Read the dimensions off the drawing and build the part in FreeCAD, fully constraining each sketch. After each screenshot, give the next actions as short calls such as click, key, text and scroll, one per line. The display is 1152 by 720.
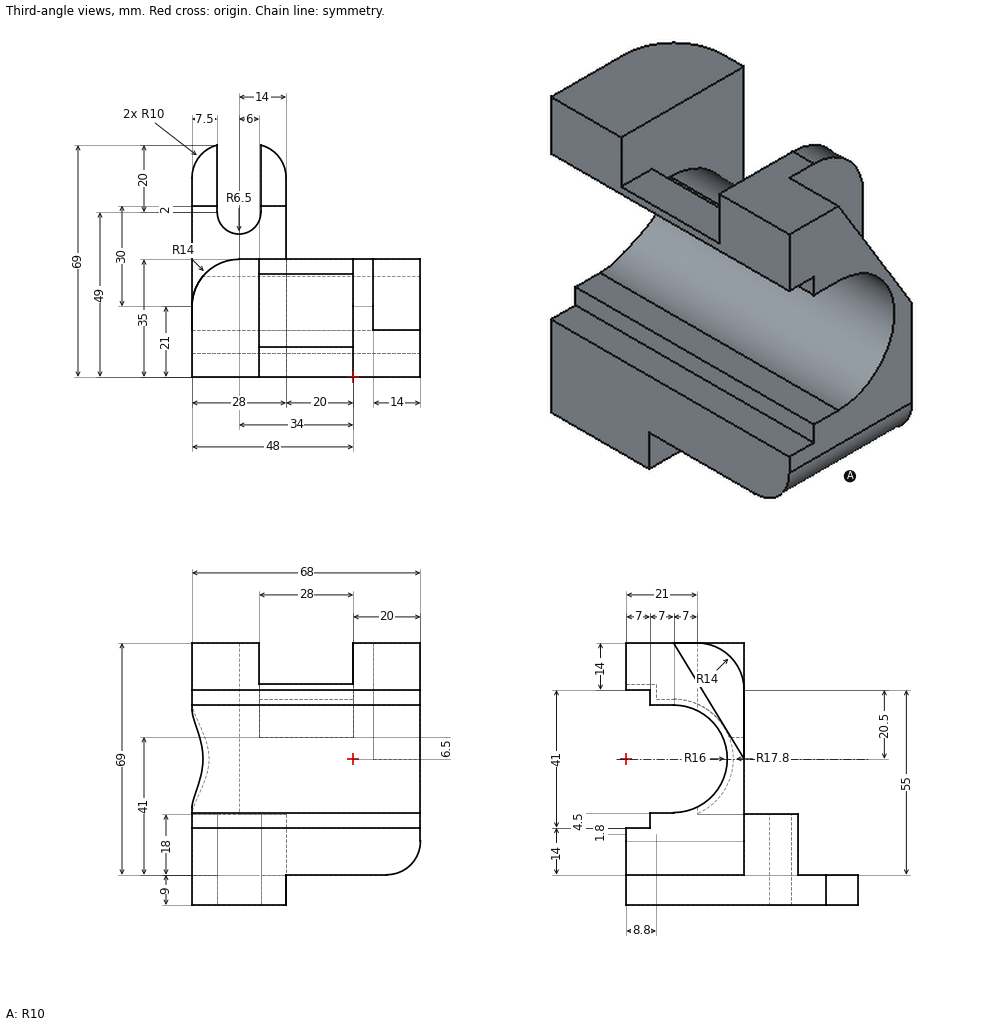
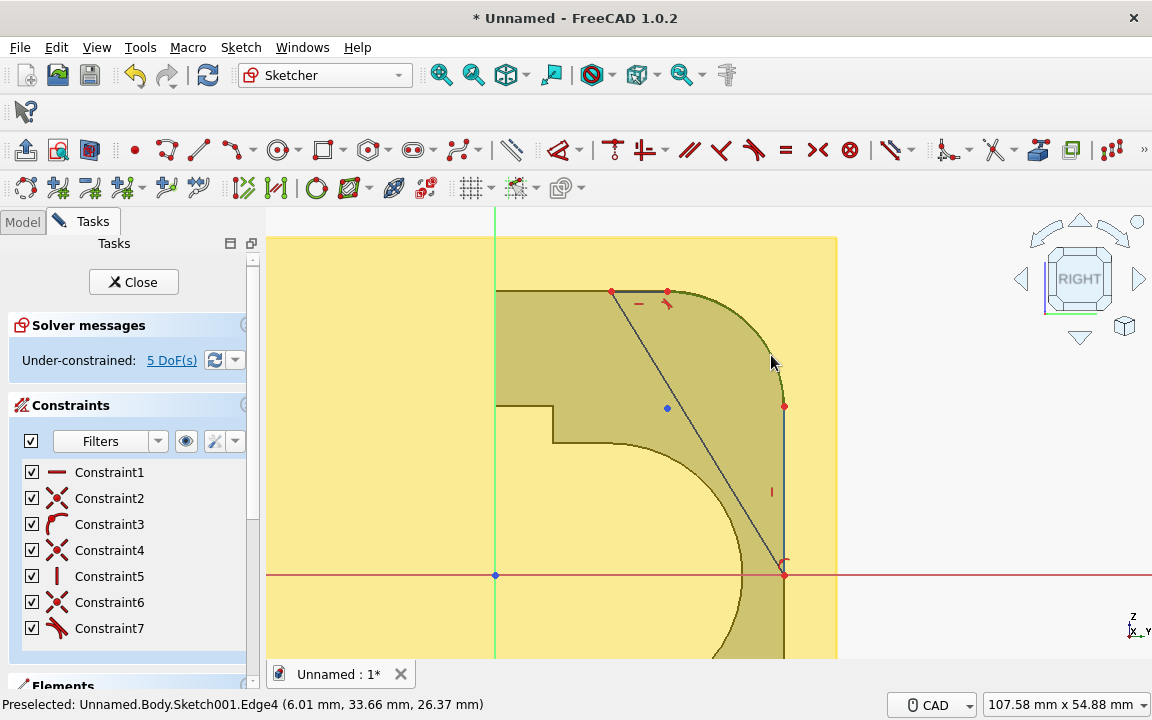
click(754, 150)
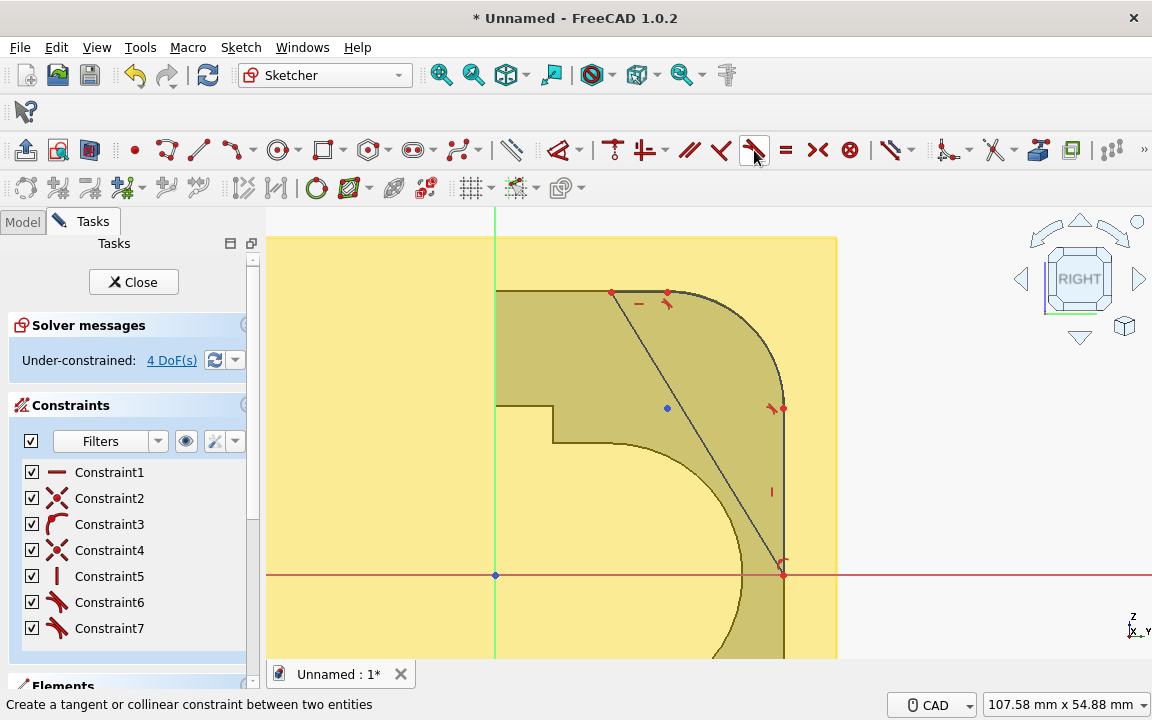
key(d)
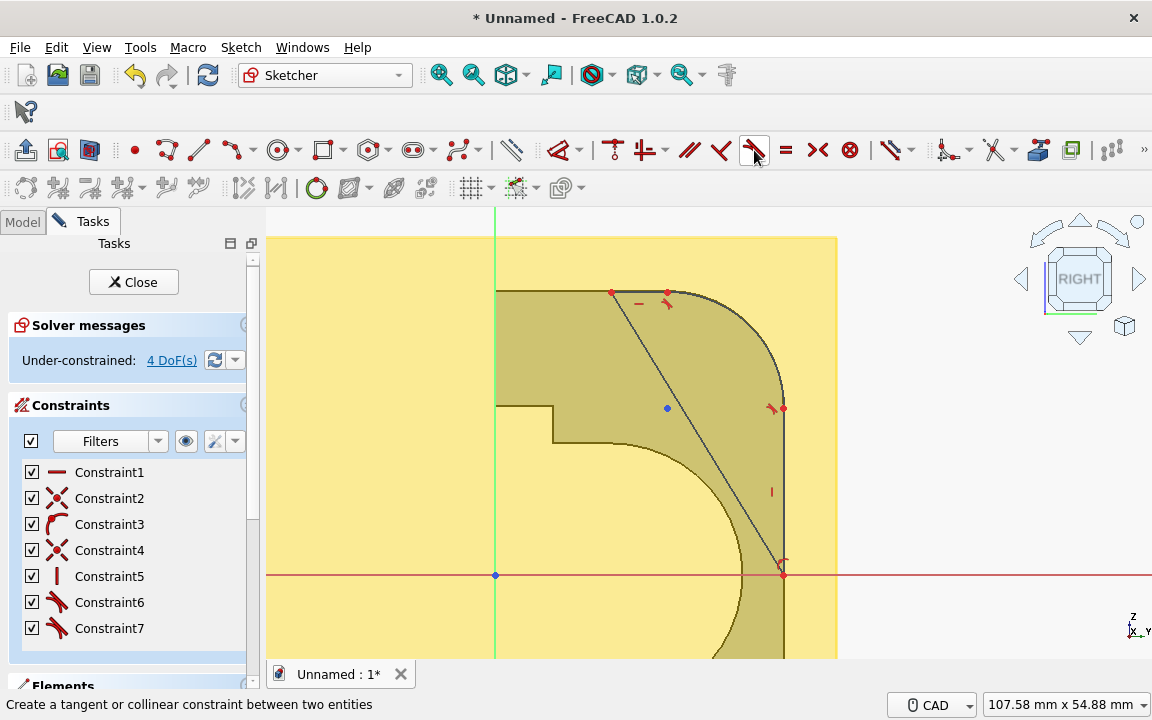
click(771, 355)
click(799, 340)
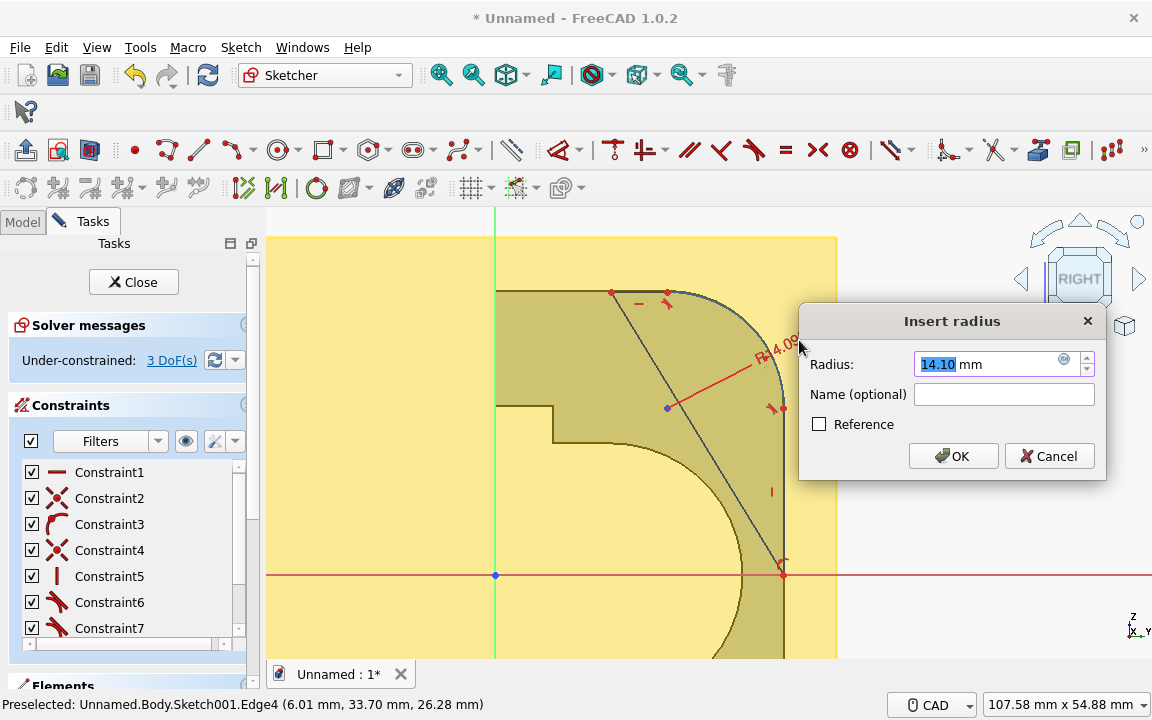
text(14)
key(Return)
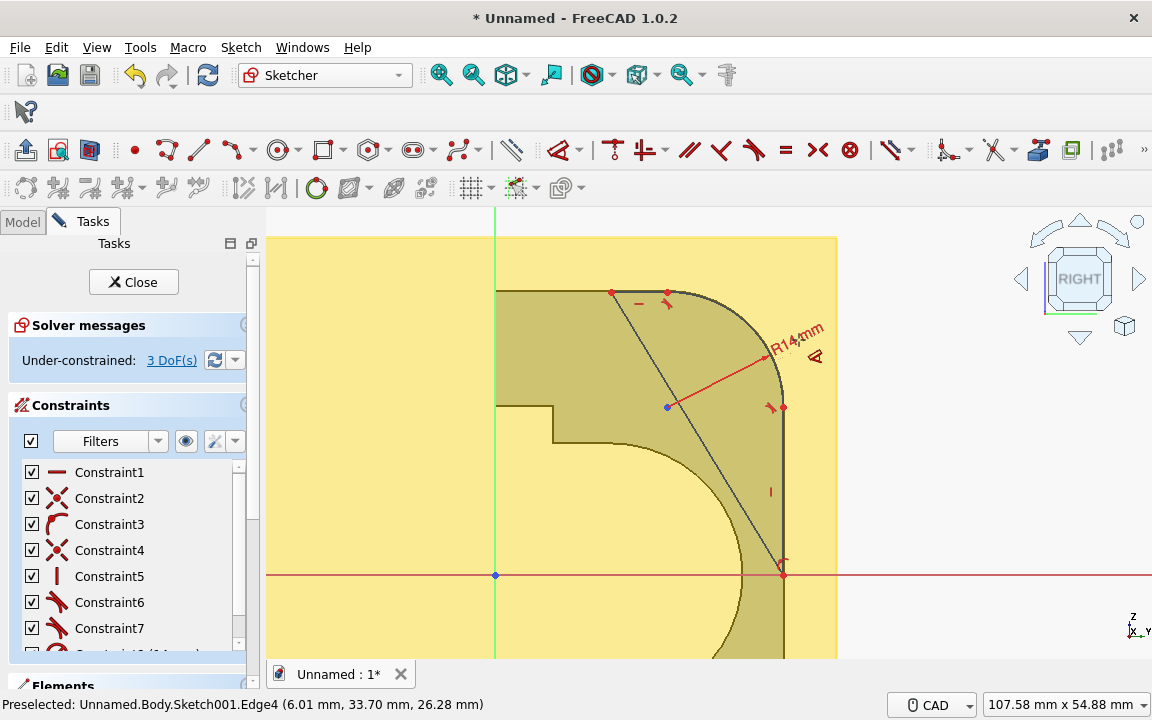
click(651, 292)
click(639, 258)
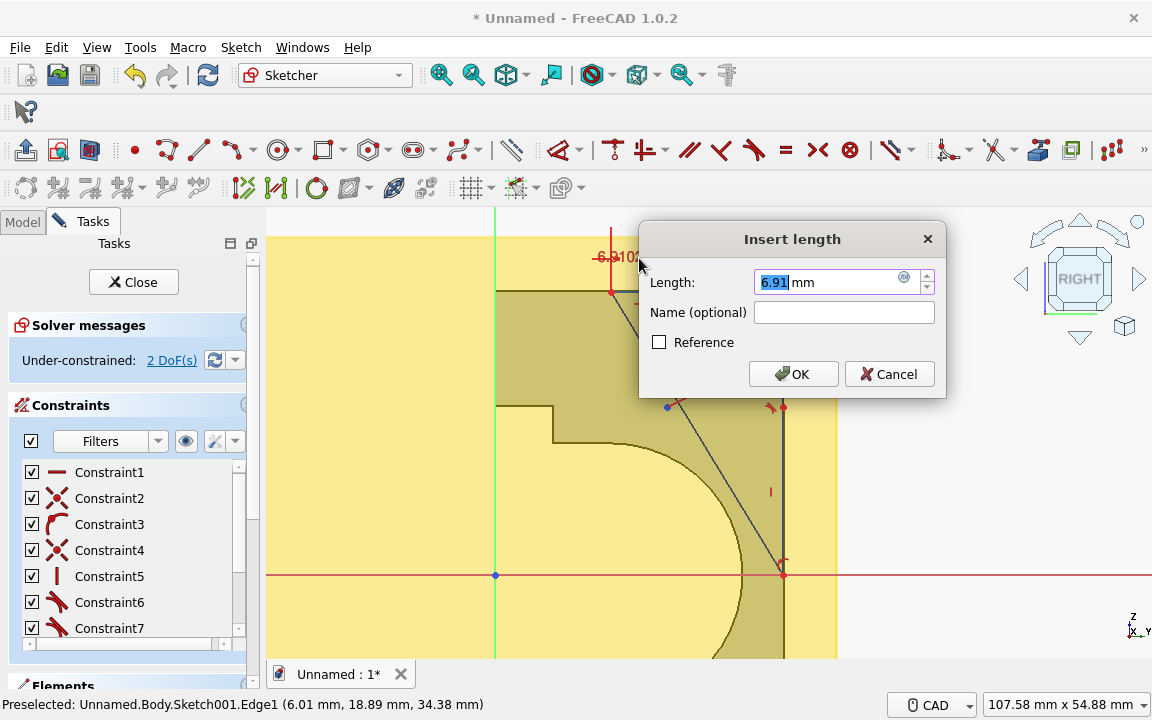
text(7)
key(Return)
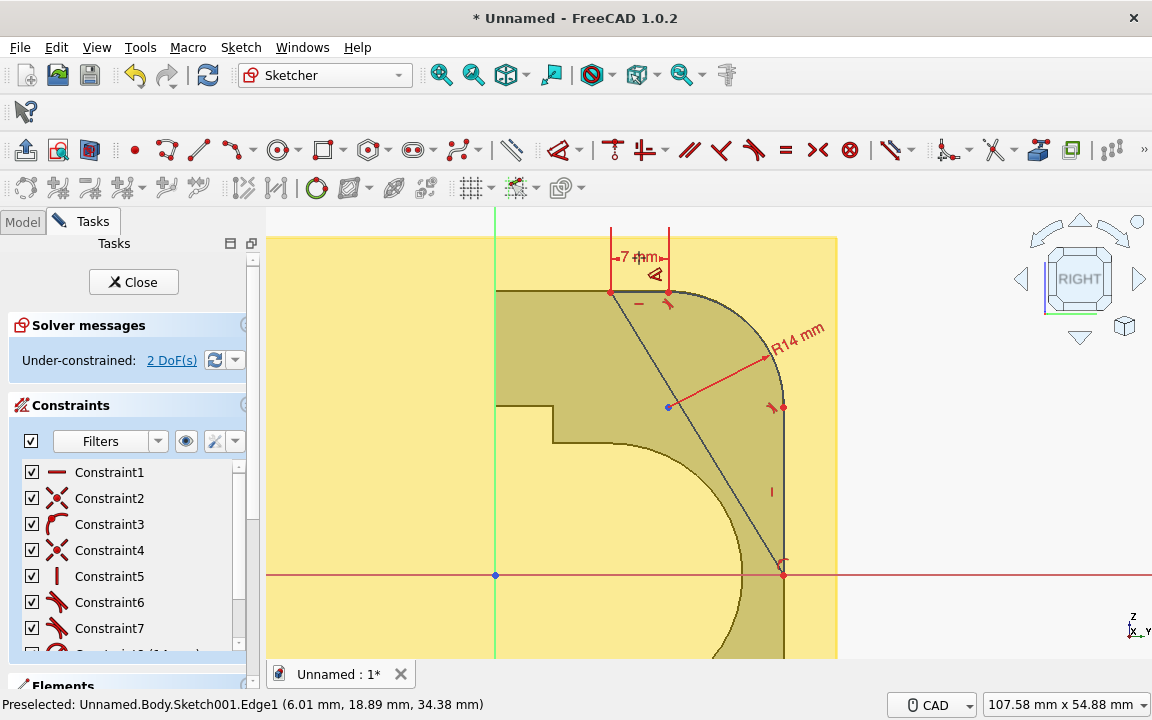
click(669, 292)
click(582, 609)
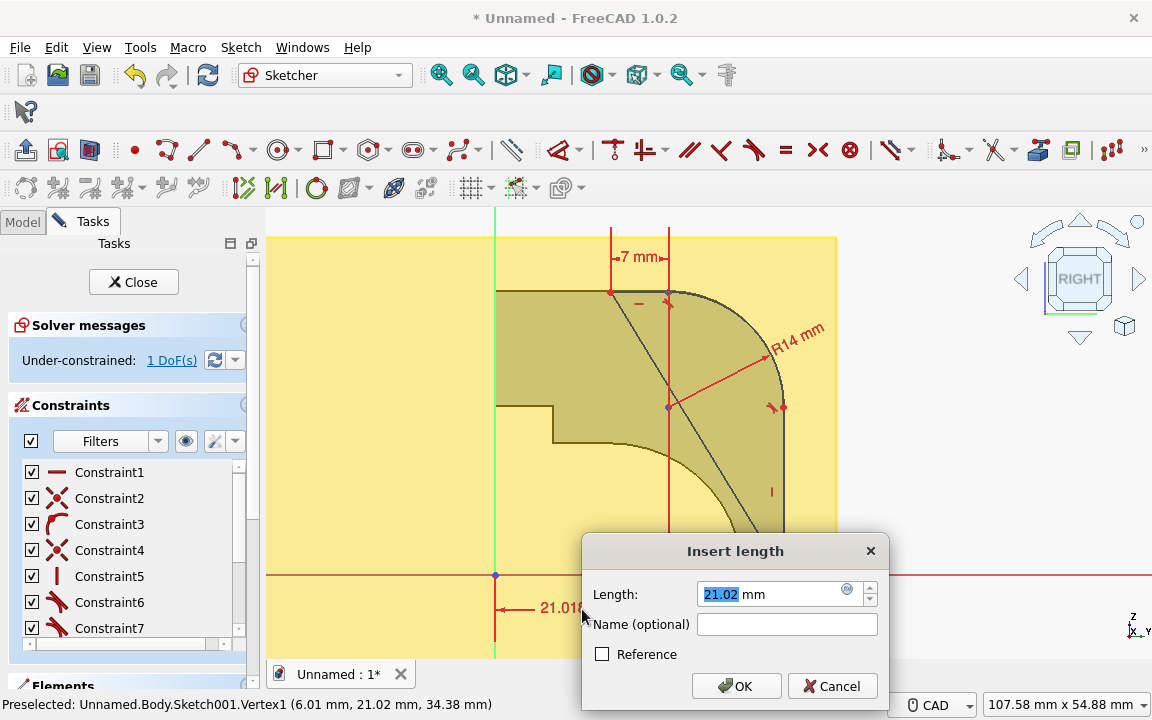
text(21)
key(Return)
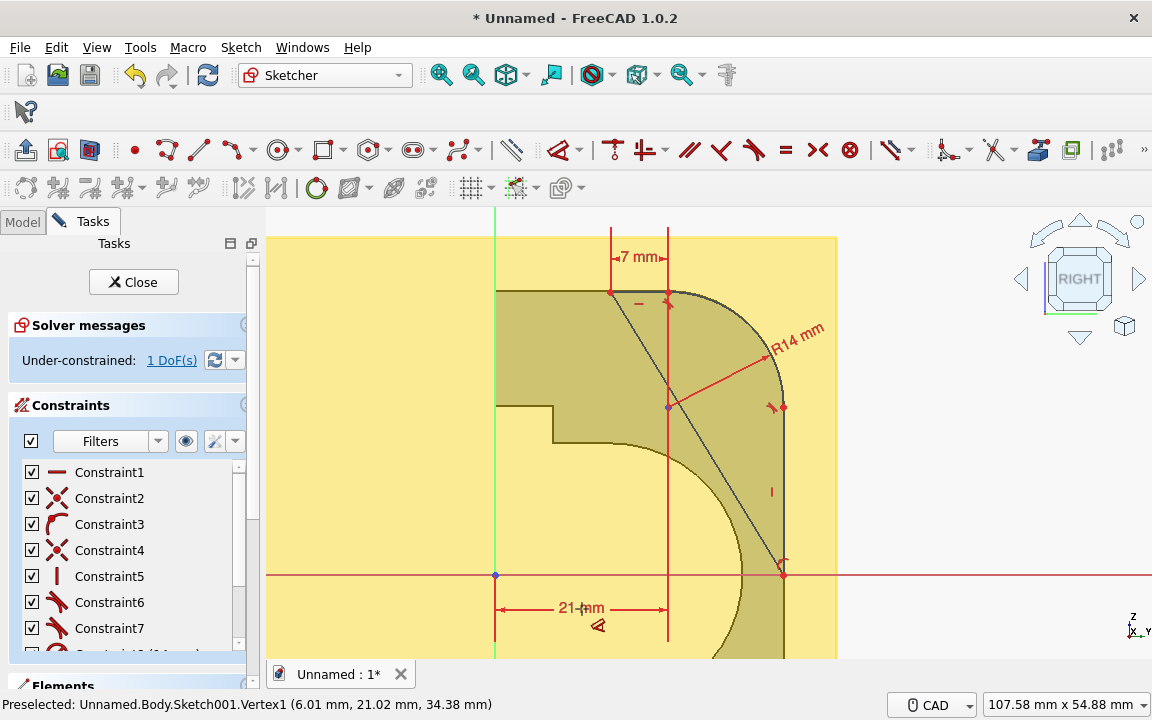
click(784, 525)
click(818, 491)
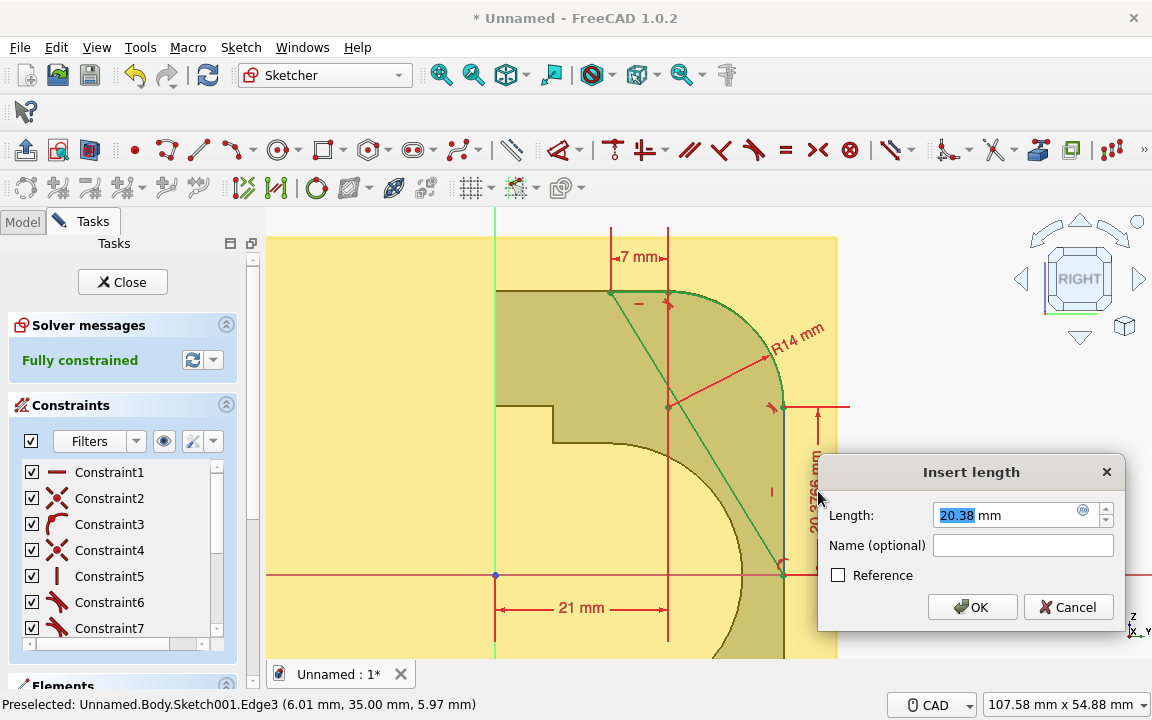
text(20.5)
key(Return)
key(Escape)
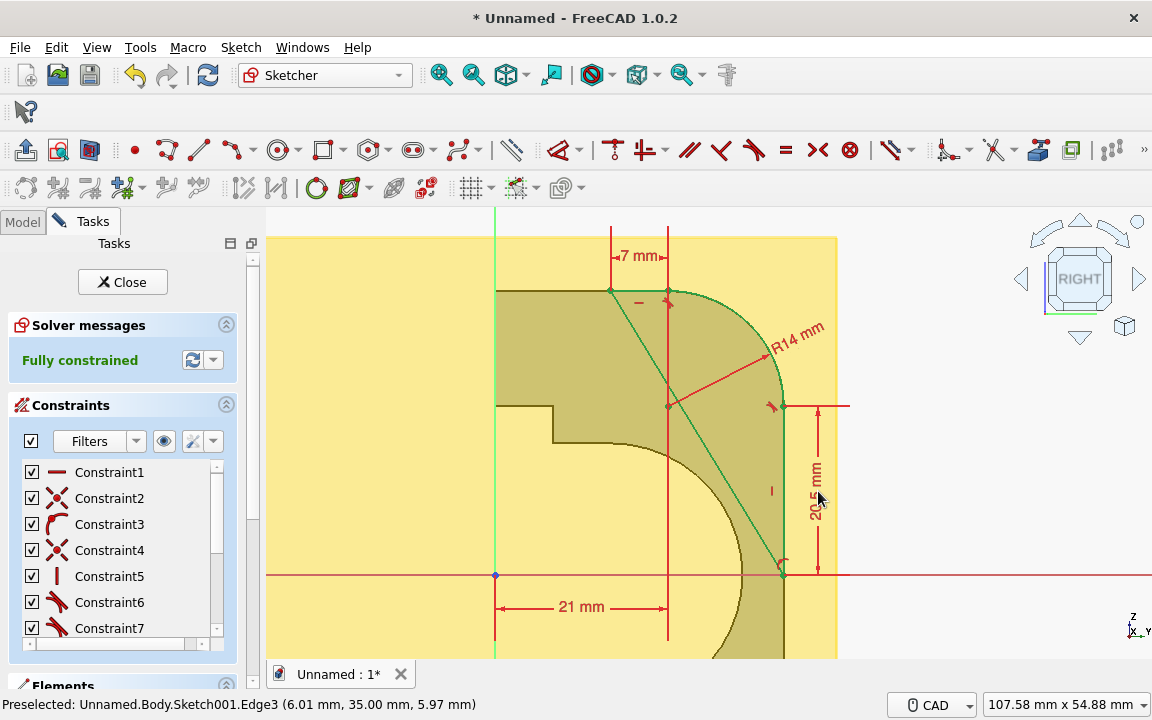
click(123, 282)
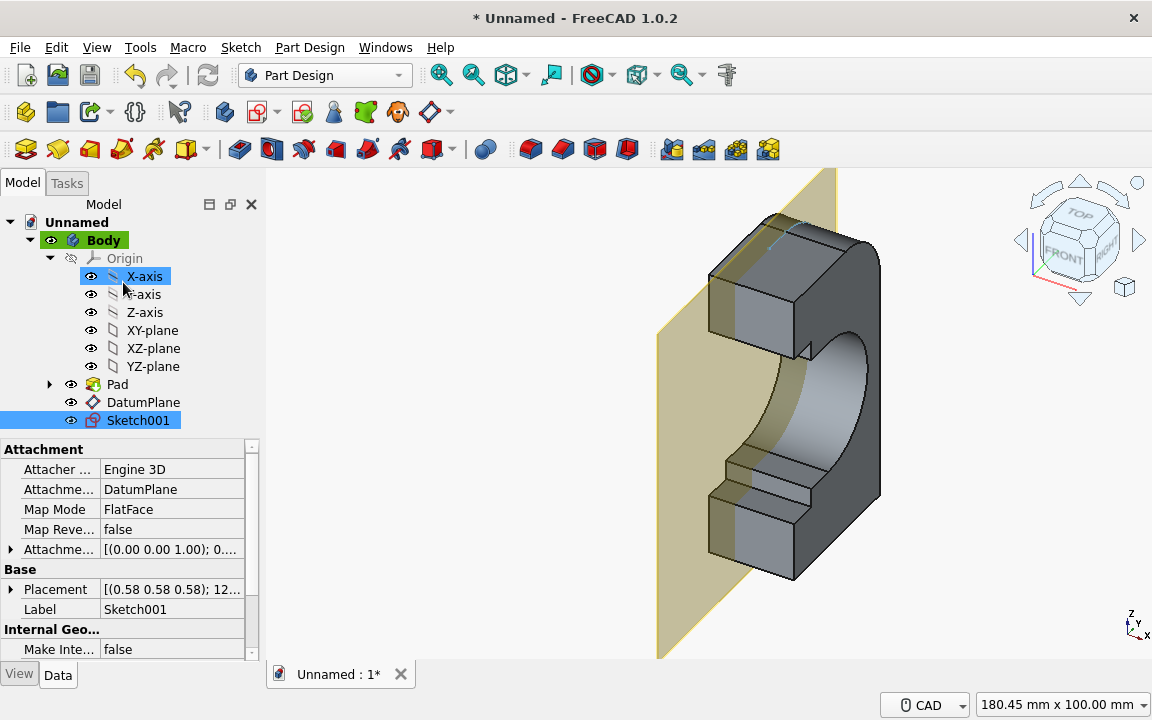
click(240, 150)